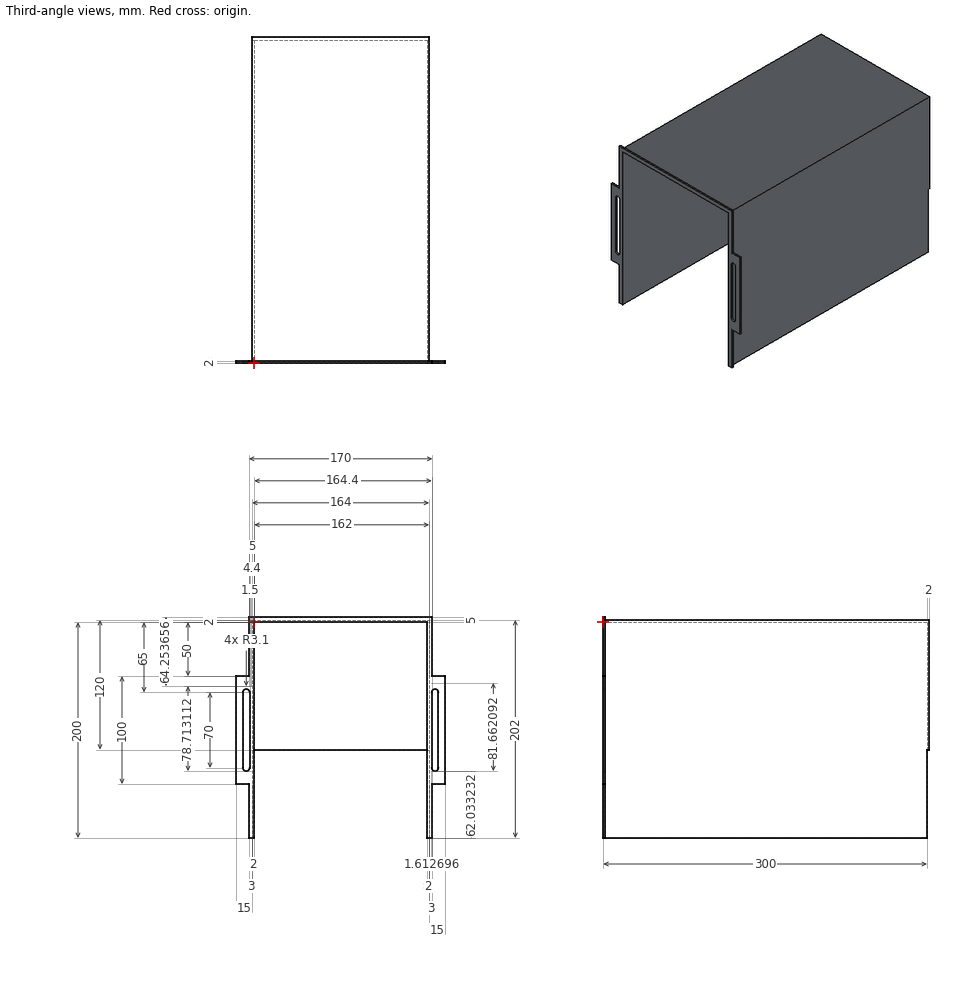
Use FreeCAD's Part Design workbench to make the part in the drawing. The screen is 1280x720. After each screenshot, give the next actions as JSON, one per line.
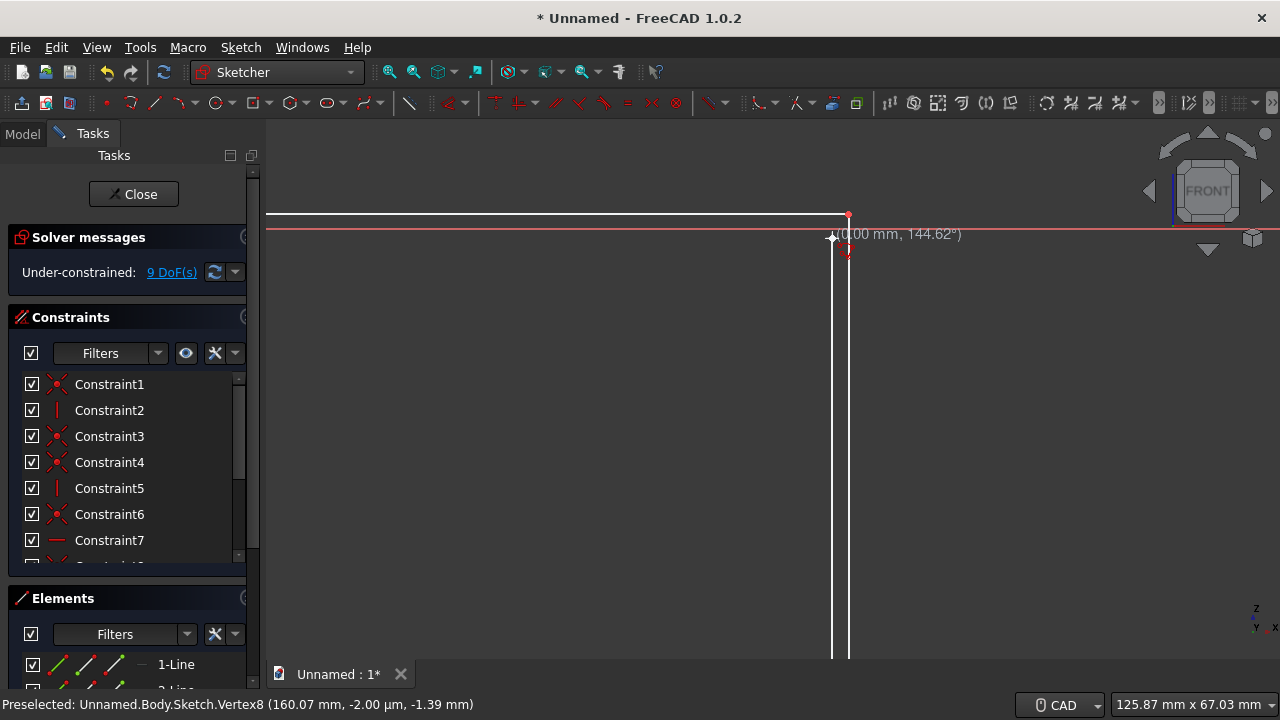
{"action": "scroll", "coordinate": [835, 228], "scroll_direction": "down", "scroll_amount": 8}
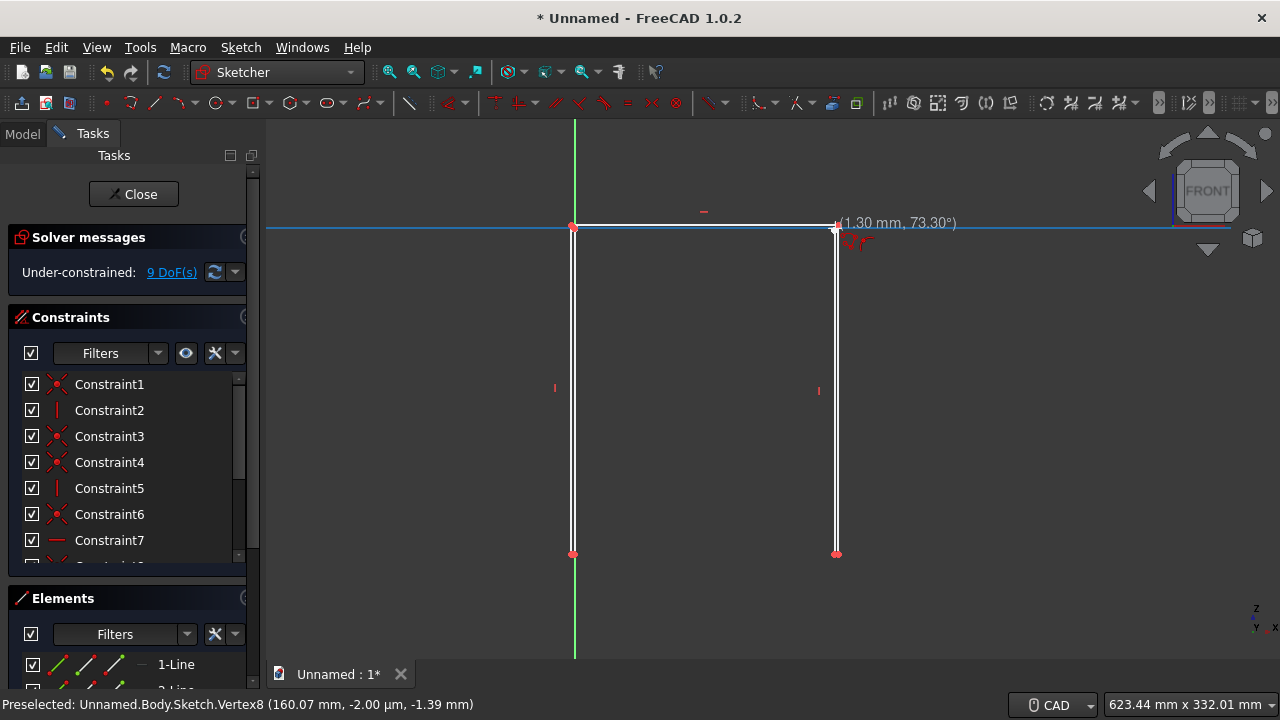
{"action": "scroll", "coordinate": [575, 228], "scroll_direction": "up", "scroll_amount": 8}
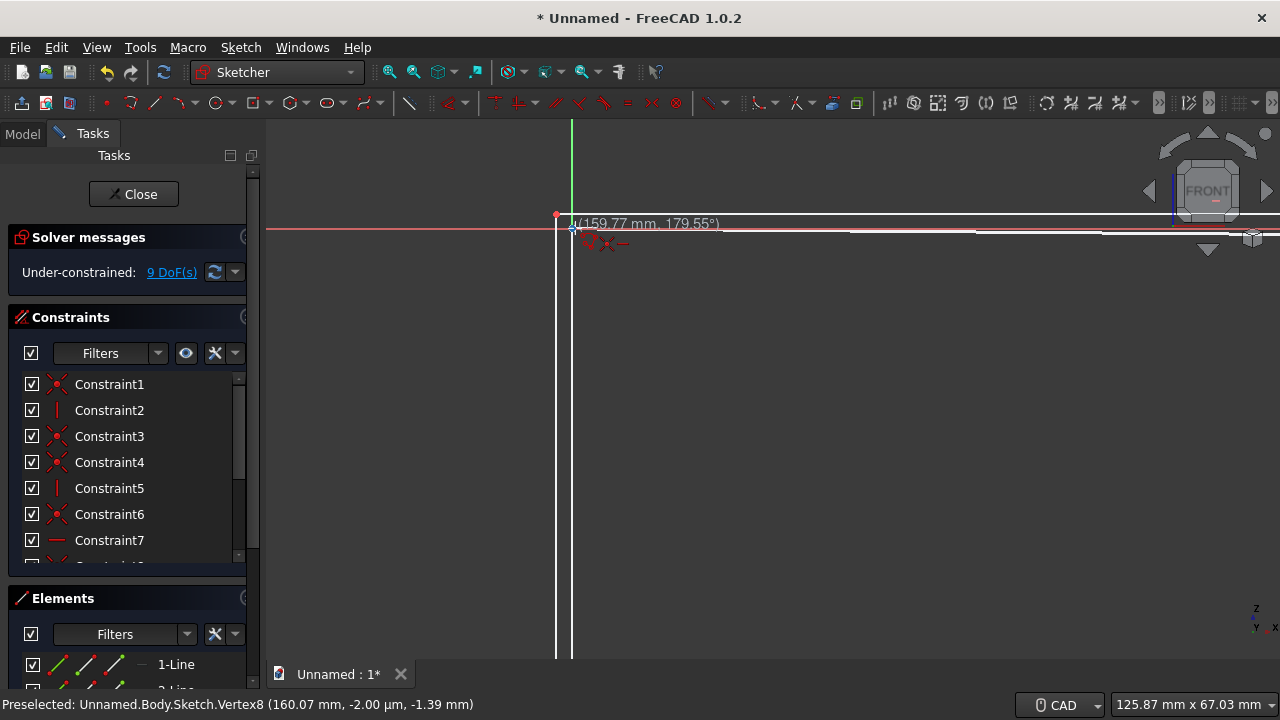
{"action": "left_click", "coordinate": [572, 229]}
{"action": "key", "text": "Escape"}
{"action": "key", "text": "Escape"}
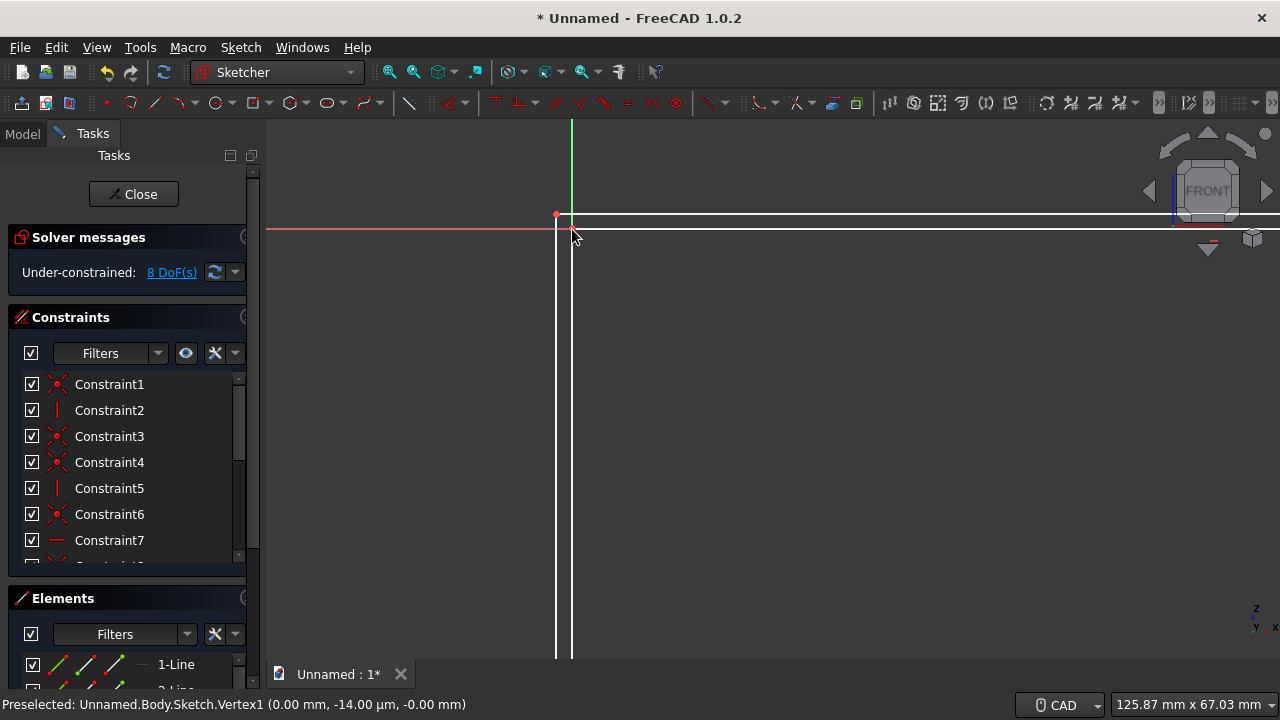
{"action": "scroll", "coordinate": [575, 228], "scroll_direction": "down", "scroll_amount": 8}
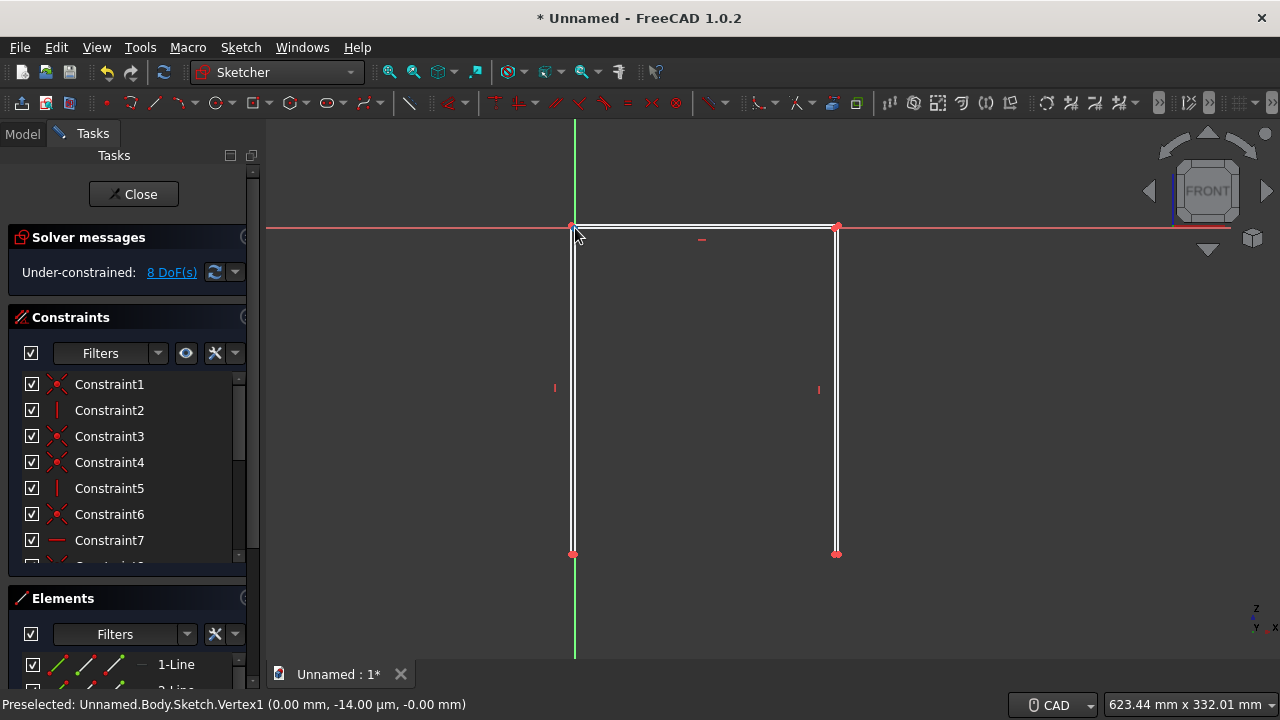
{"action": "scroll", "coordinate": [573, 555], "scroll_direction": "up", "scroll_amount": 11}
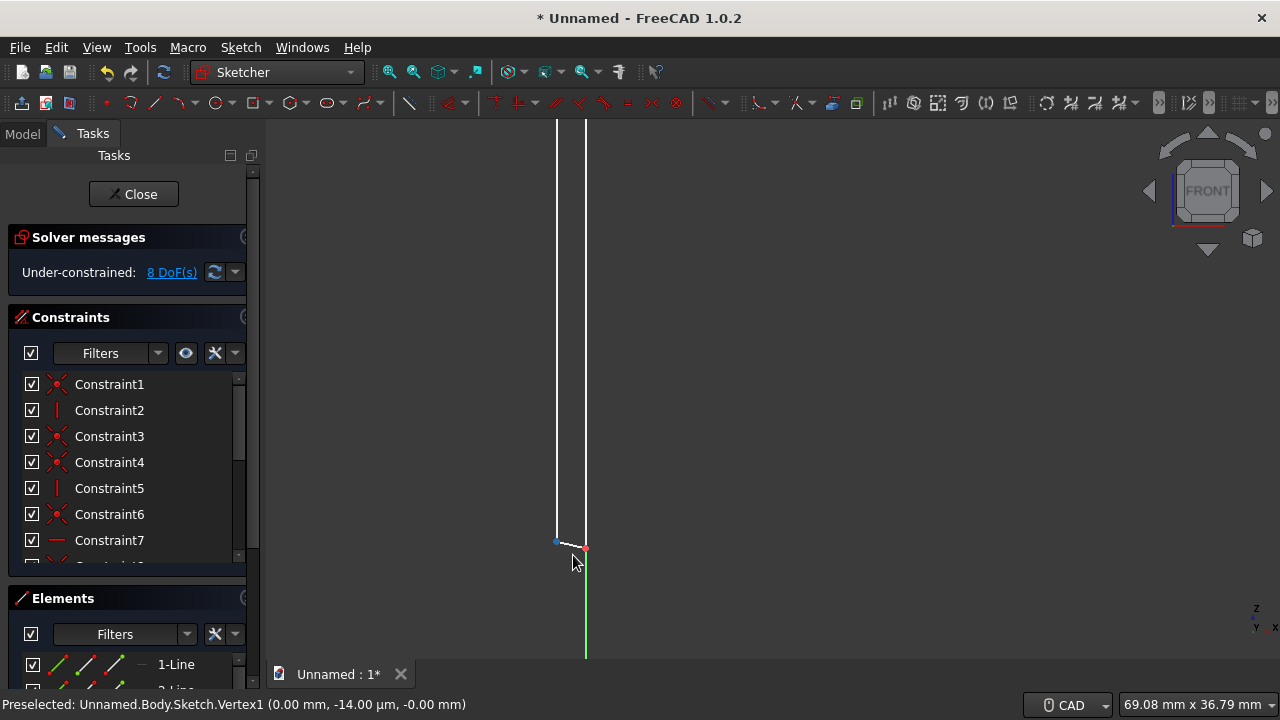
{"action": "left_click", "coordinate": [571, 545]}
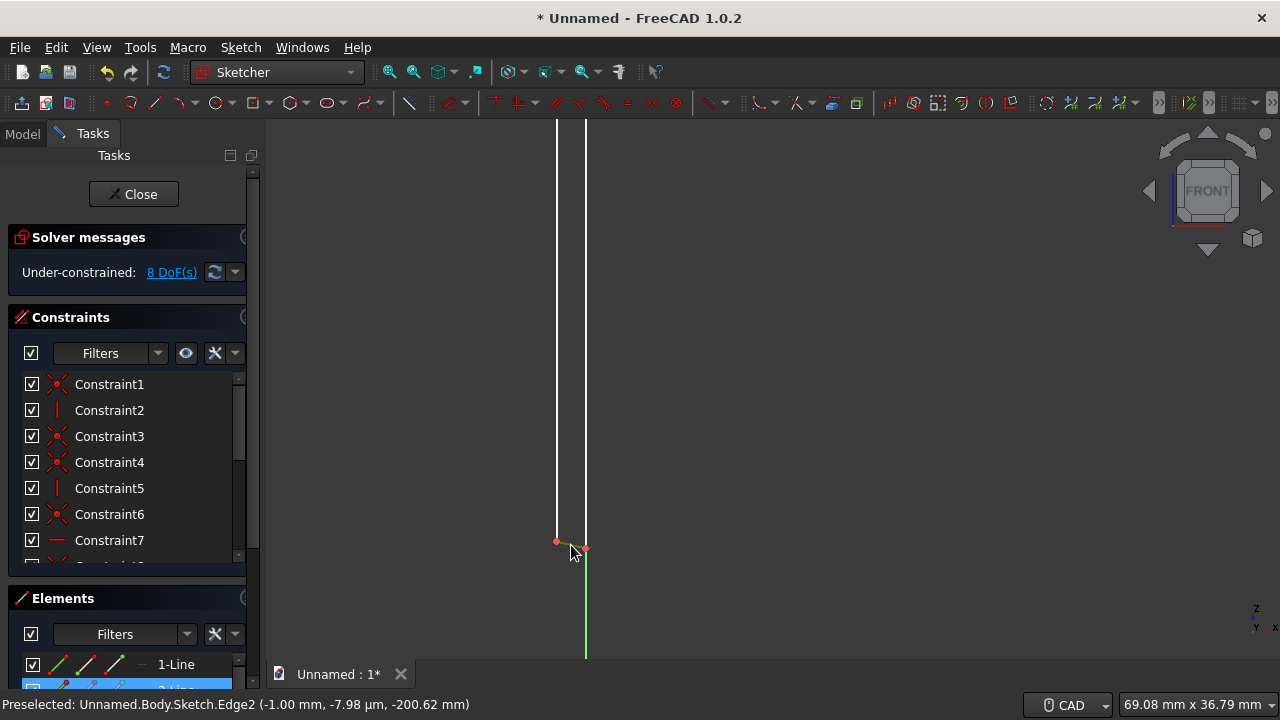
{"action": "left_click", "coordinate": [538, 104]}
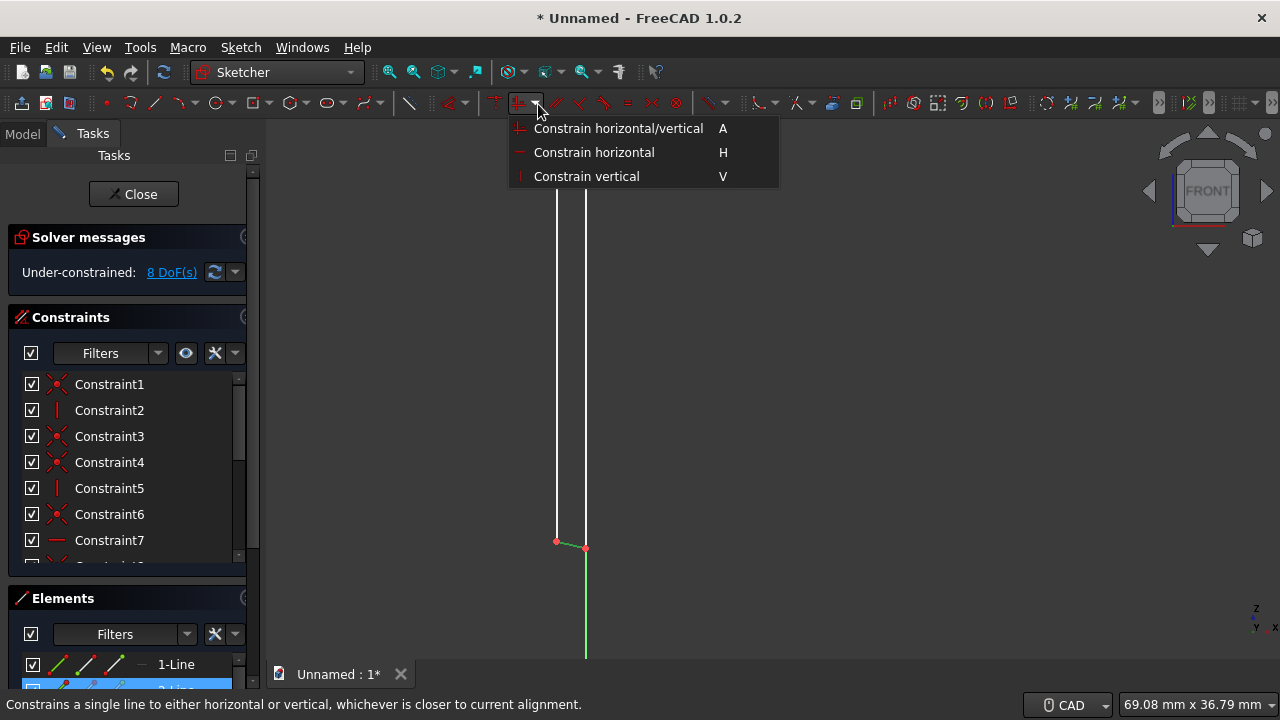
{"action": "left_click", "coordinate": [644, 152]}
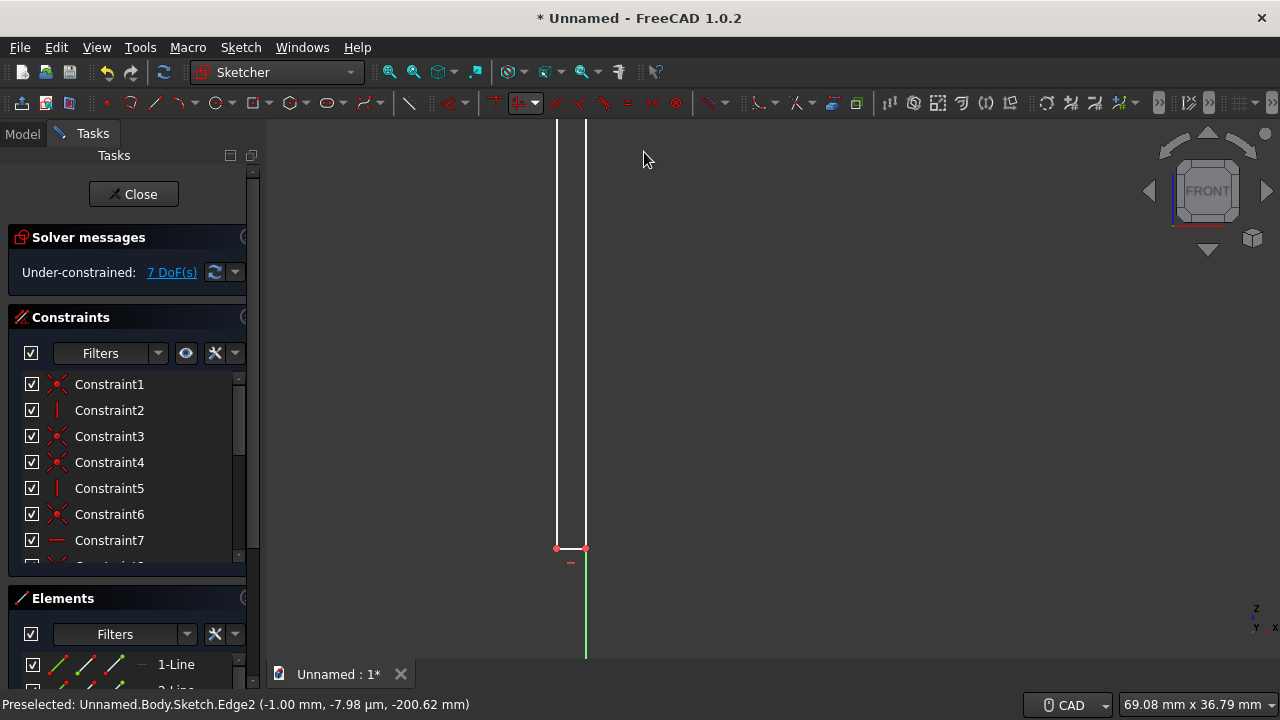
{"action": "scroll", "coordinate": [573, 555], "scroll_direction": "down", "scroll_amount": 11}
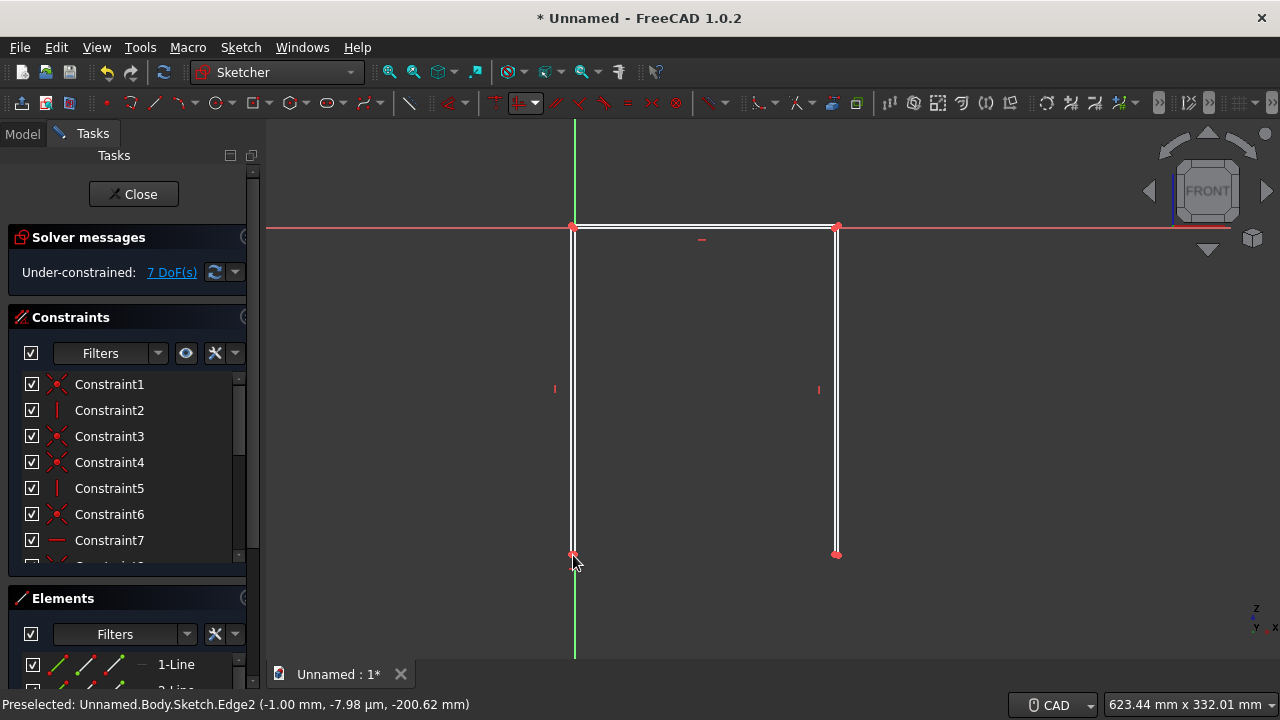
{"action": "scroll", "coordinate": [837, 555], "scroll_direction": "up", "scroll_amount": 14}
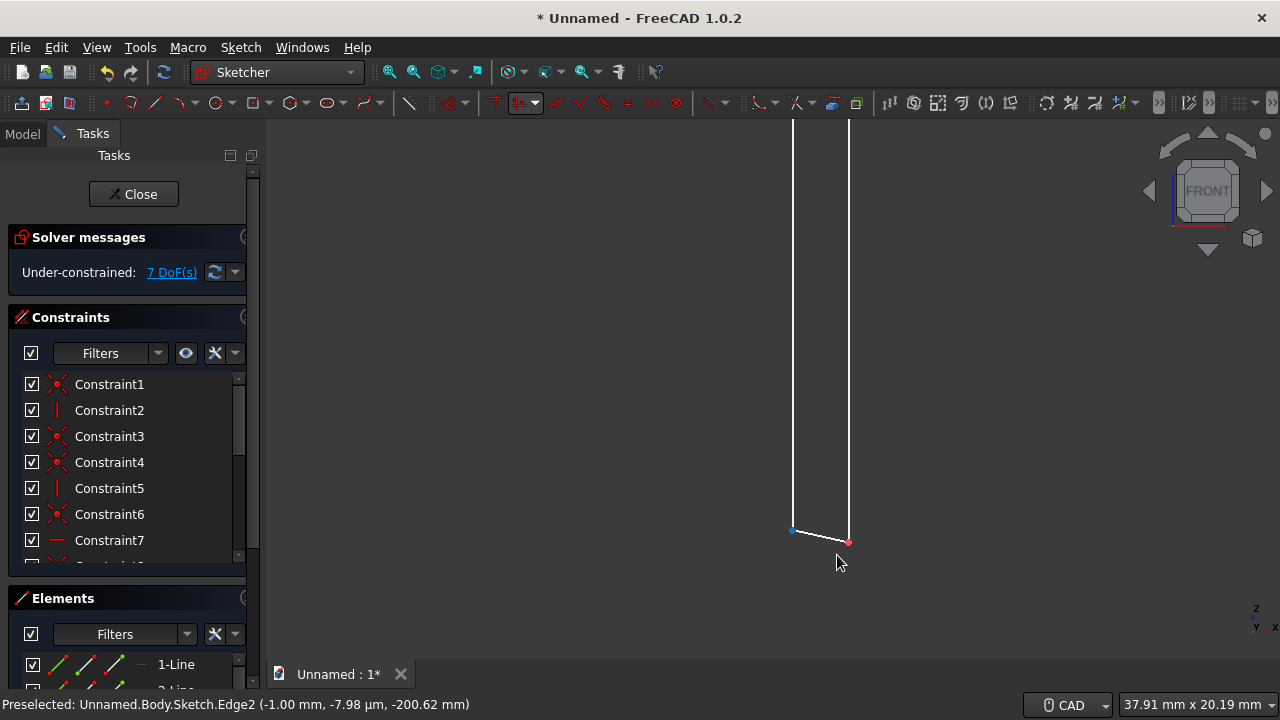
{"action": "left_click", "coordinate": [832, 539]}